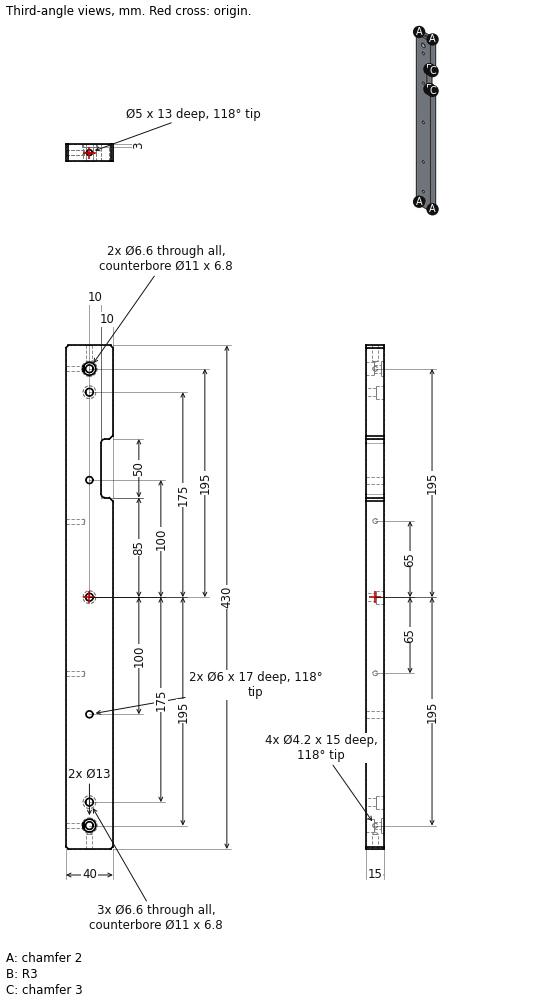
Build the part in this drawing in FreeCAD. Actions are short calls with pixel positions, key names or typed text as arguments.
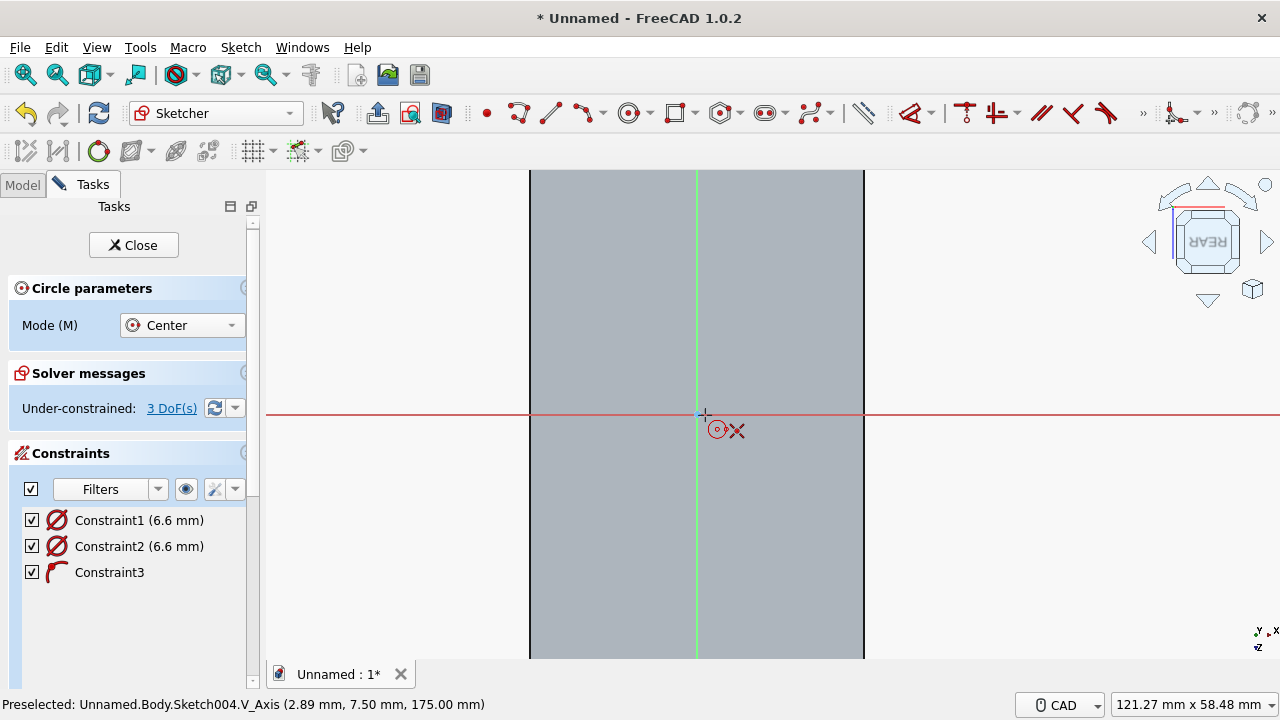
scroll(705, 415, down, 11)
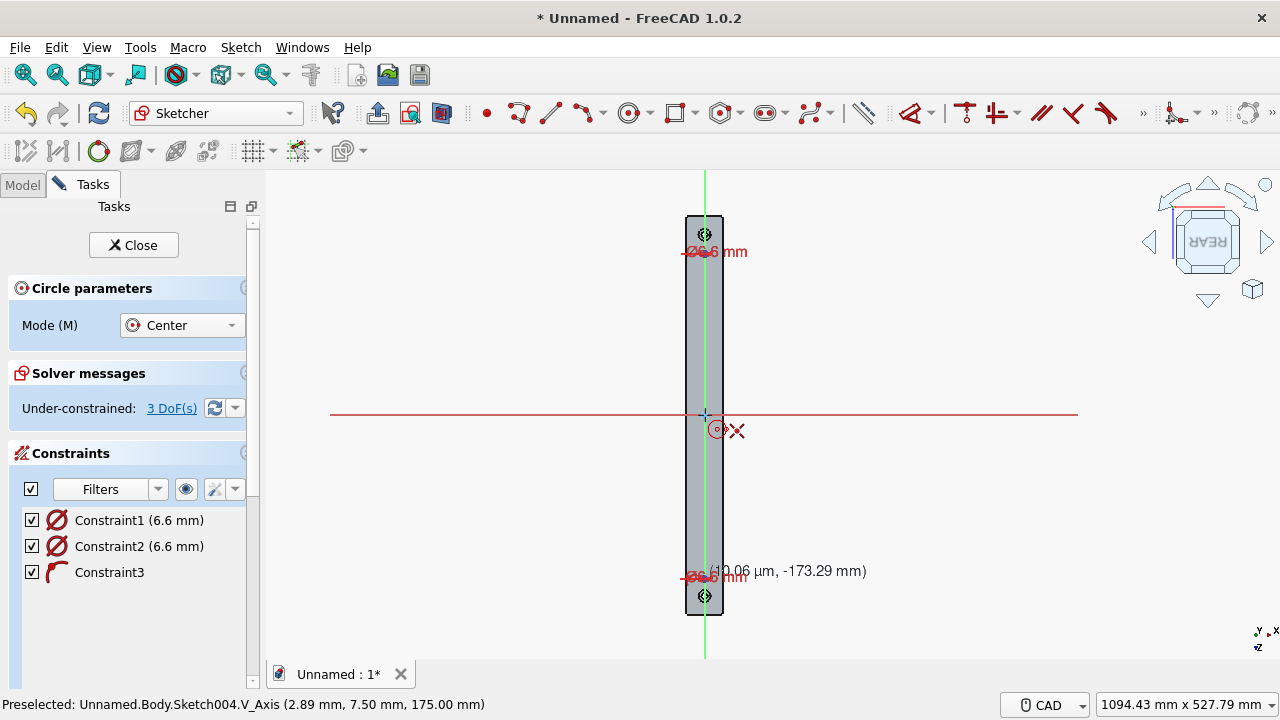
click(705, 415)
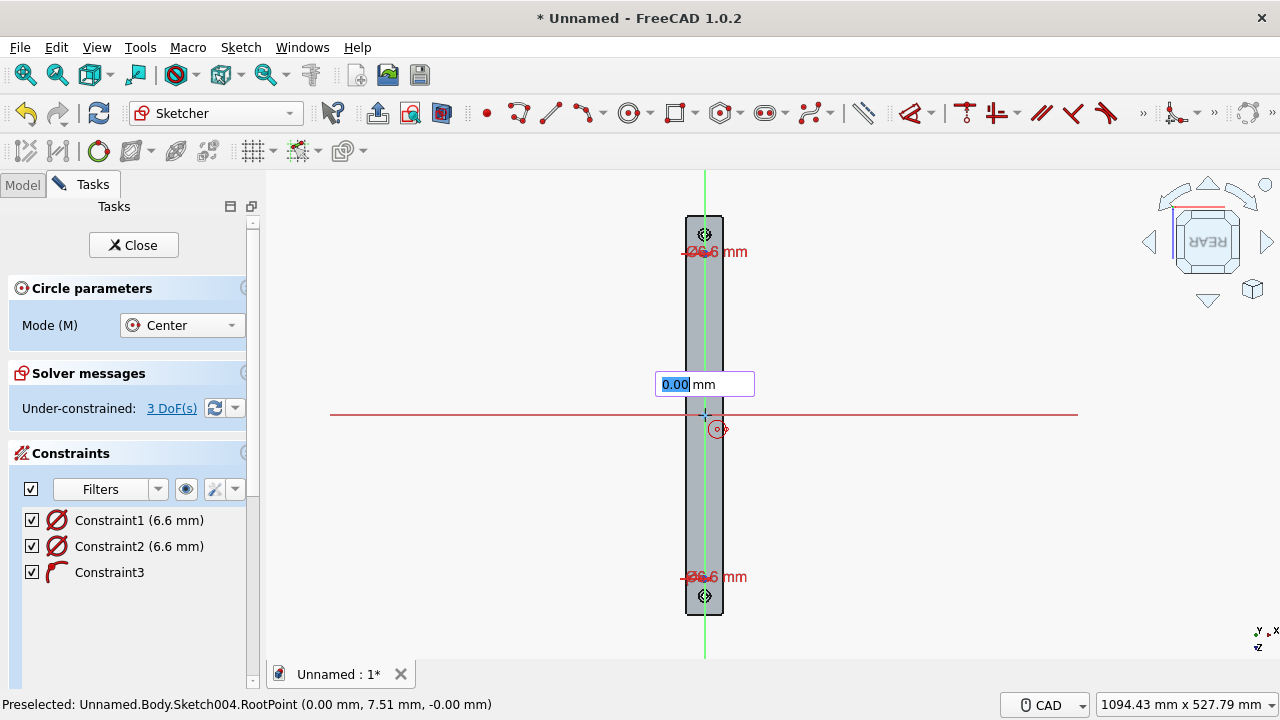
scroll(707, 413, up, 10)
move(702, 412)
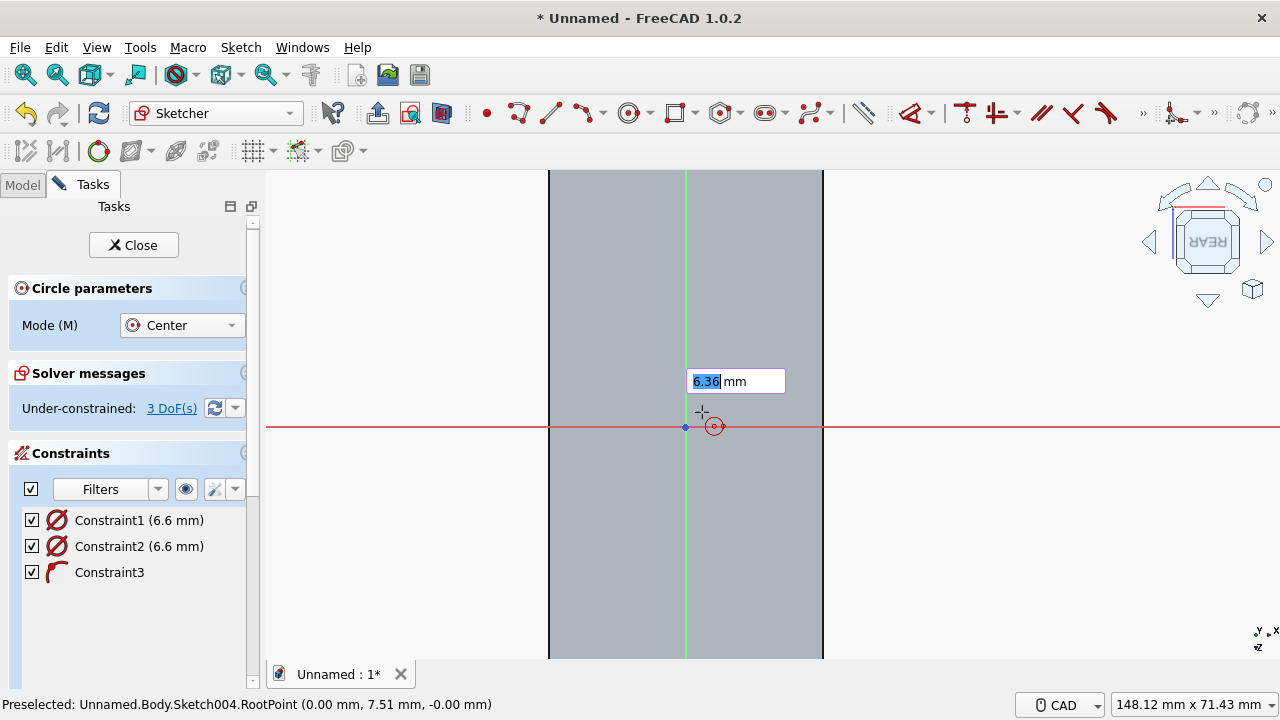
text(6.6)
key(Return)
key(Escape)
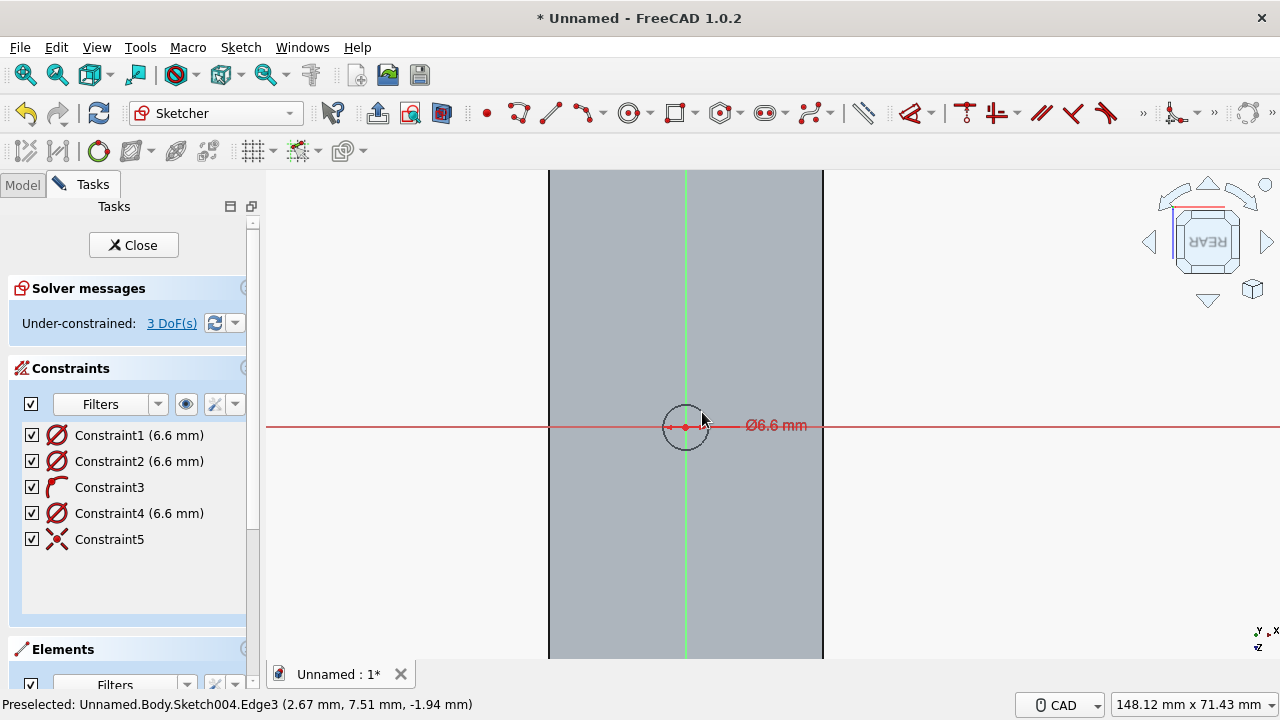
scroll(707, 412, down, 10)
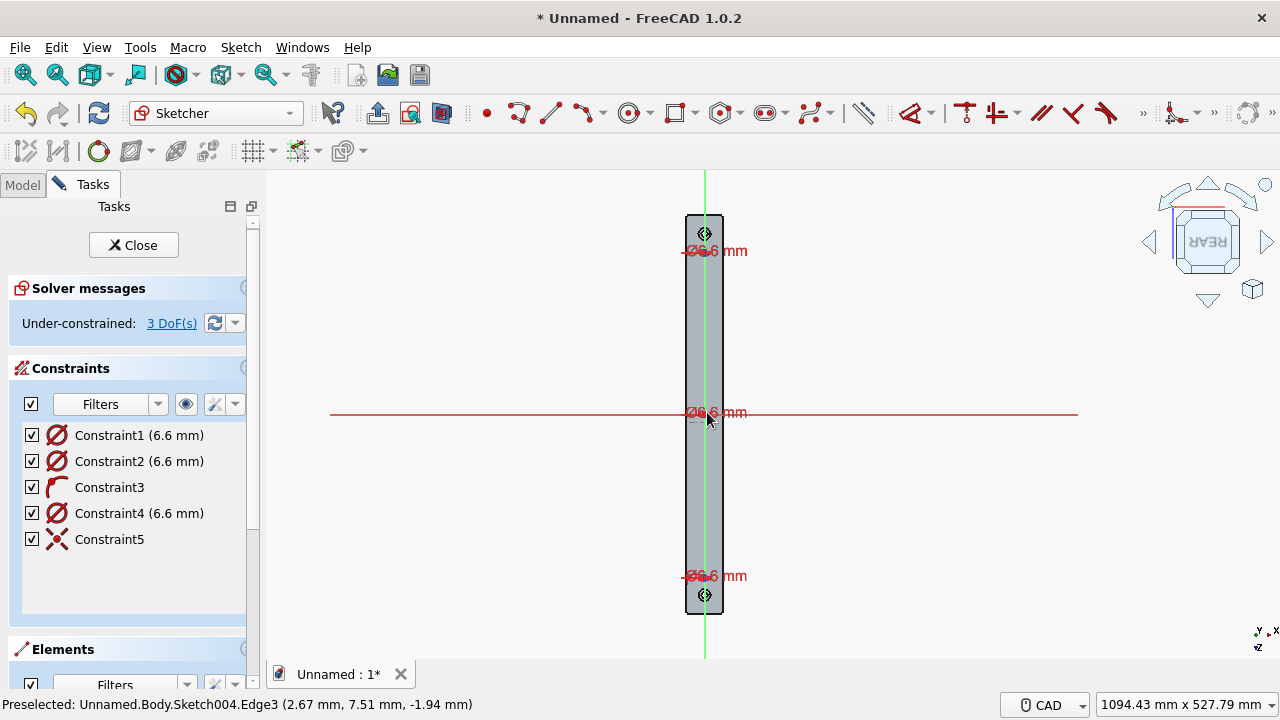
click(705, 253)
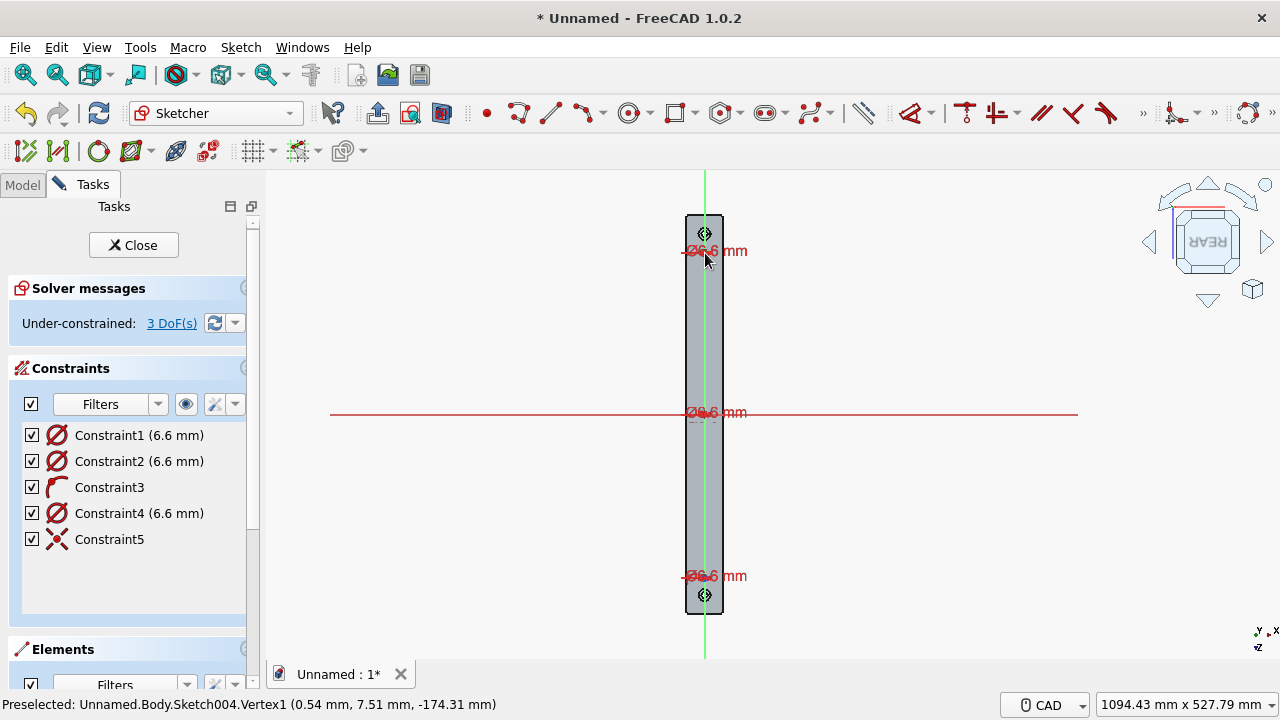
click(705, 538)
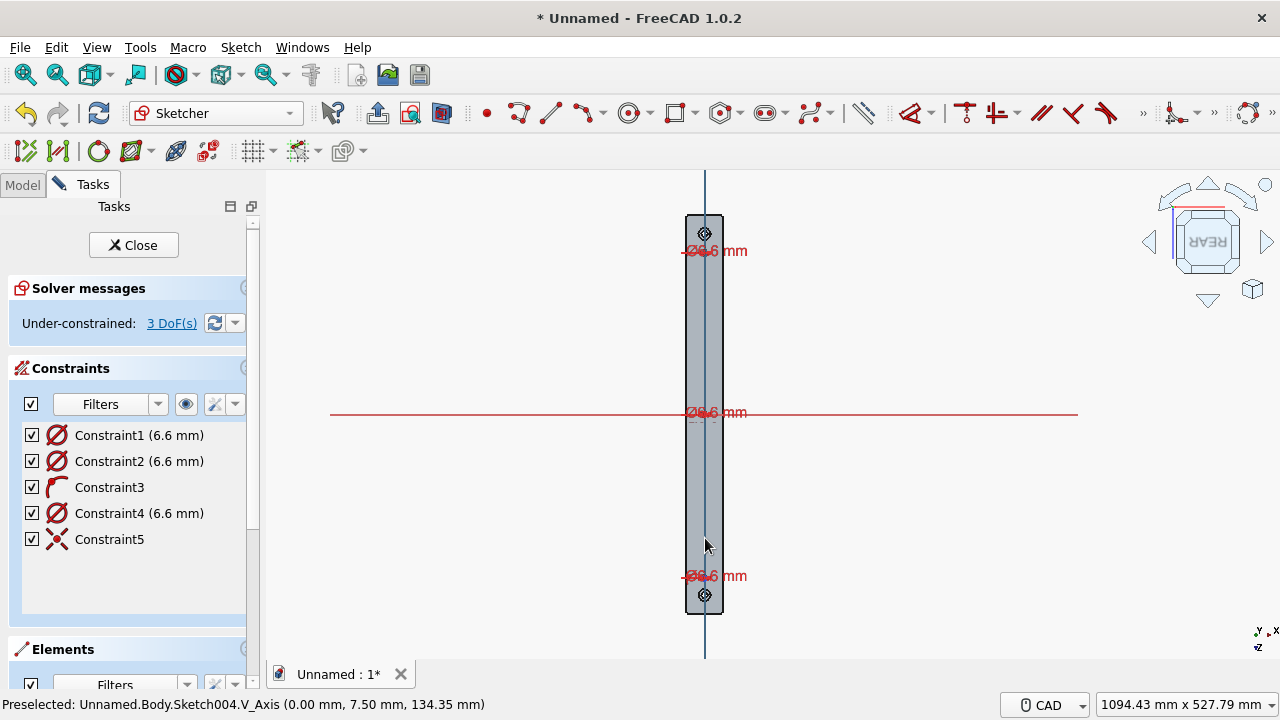
click(966, 114)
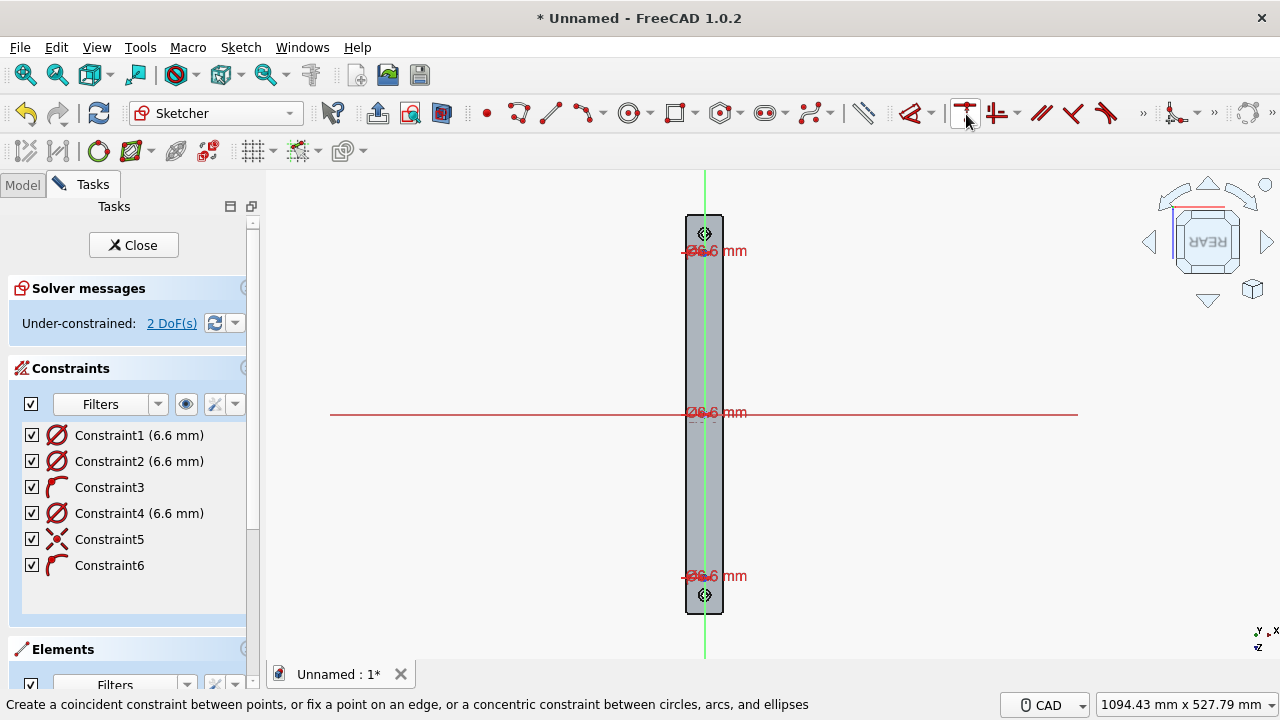
click(910, 114)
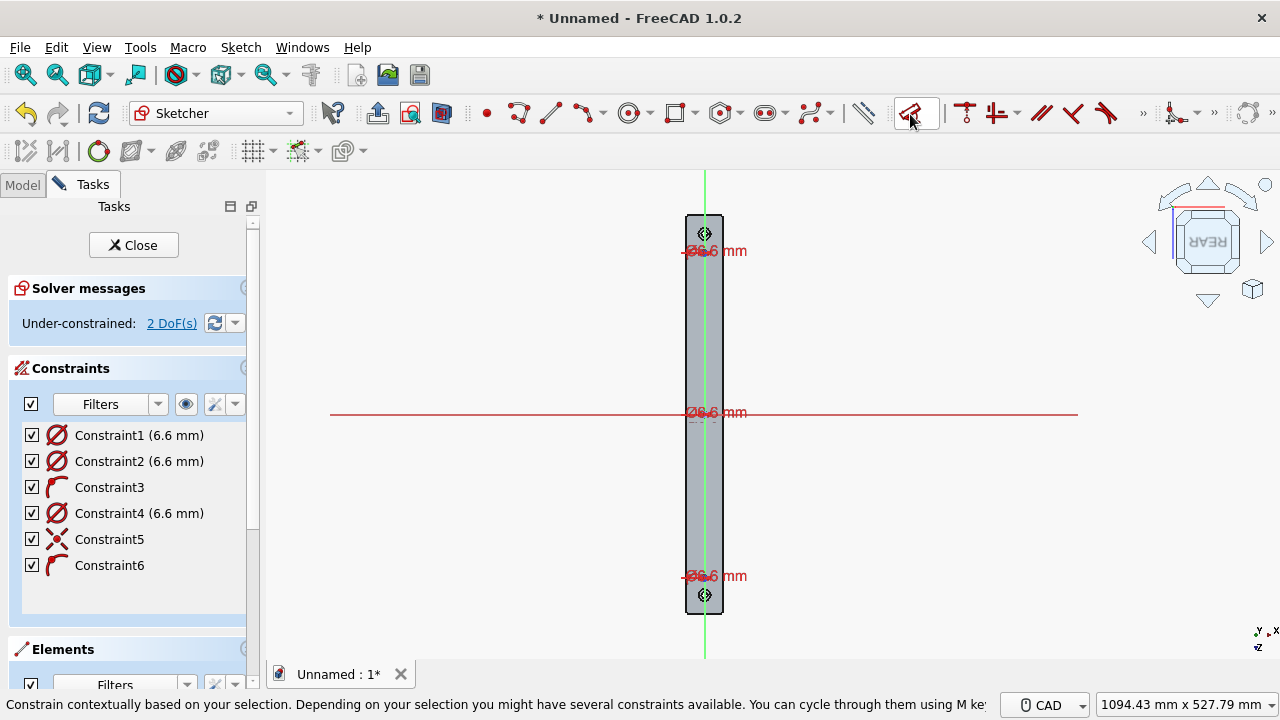
click(705, 253)
click(739, 334)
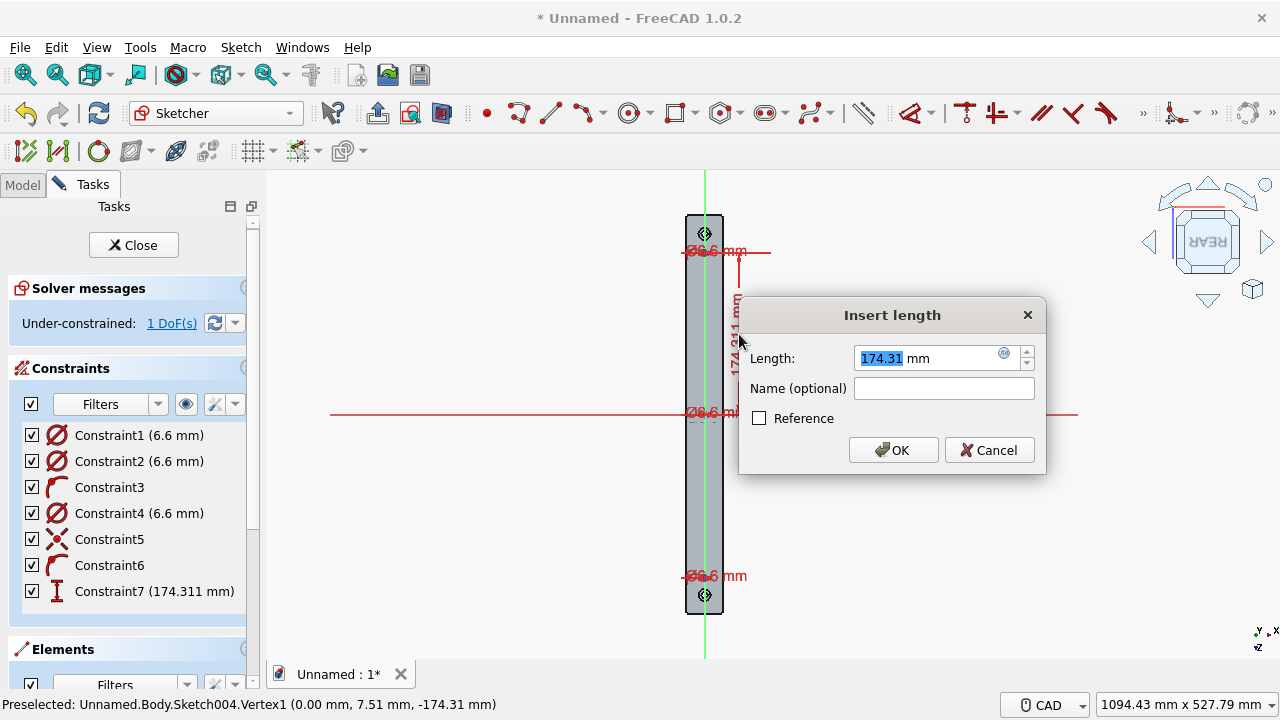
text(175)
key(Return)